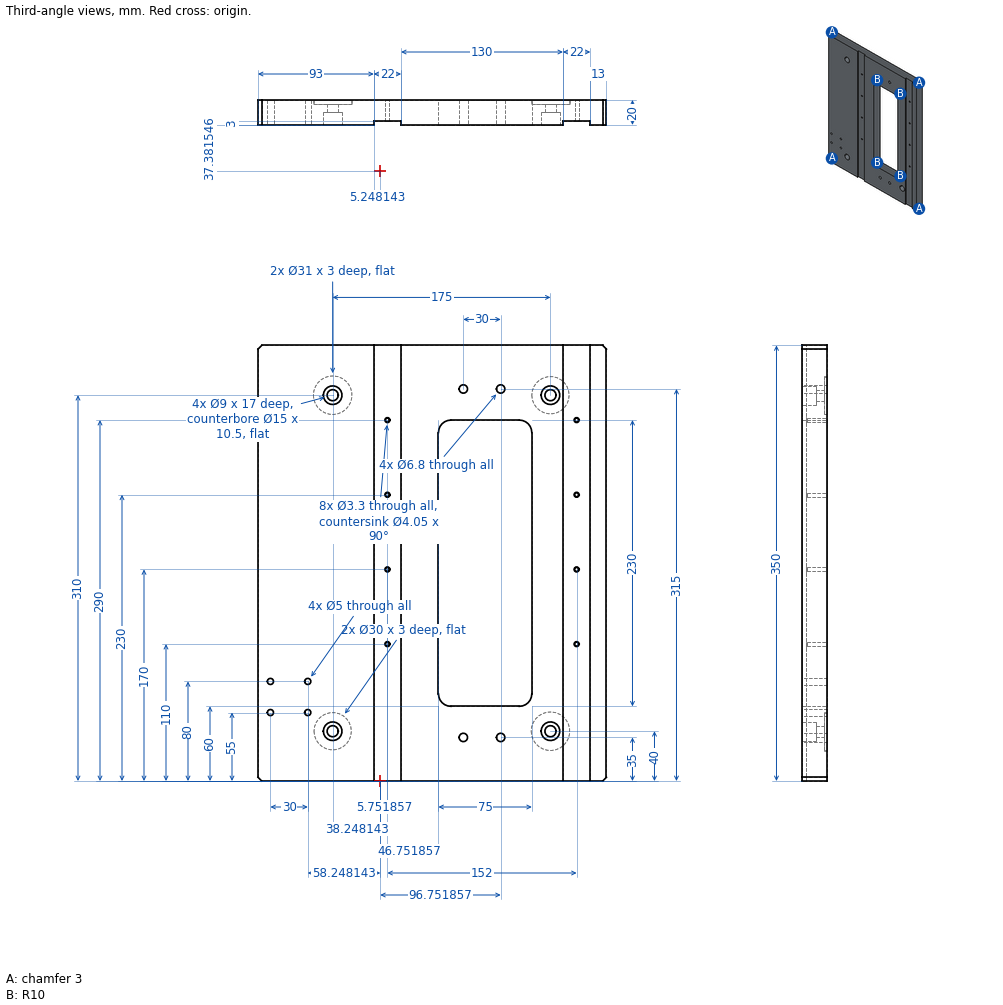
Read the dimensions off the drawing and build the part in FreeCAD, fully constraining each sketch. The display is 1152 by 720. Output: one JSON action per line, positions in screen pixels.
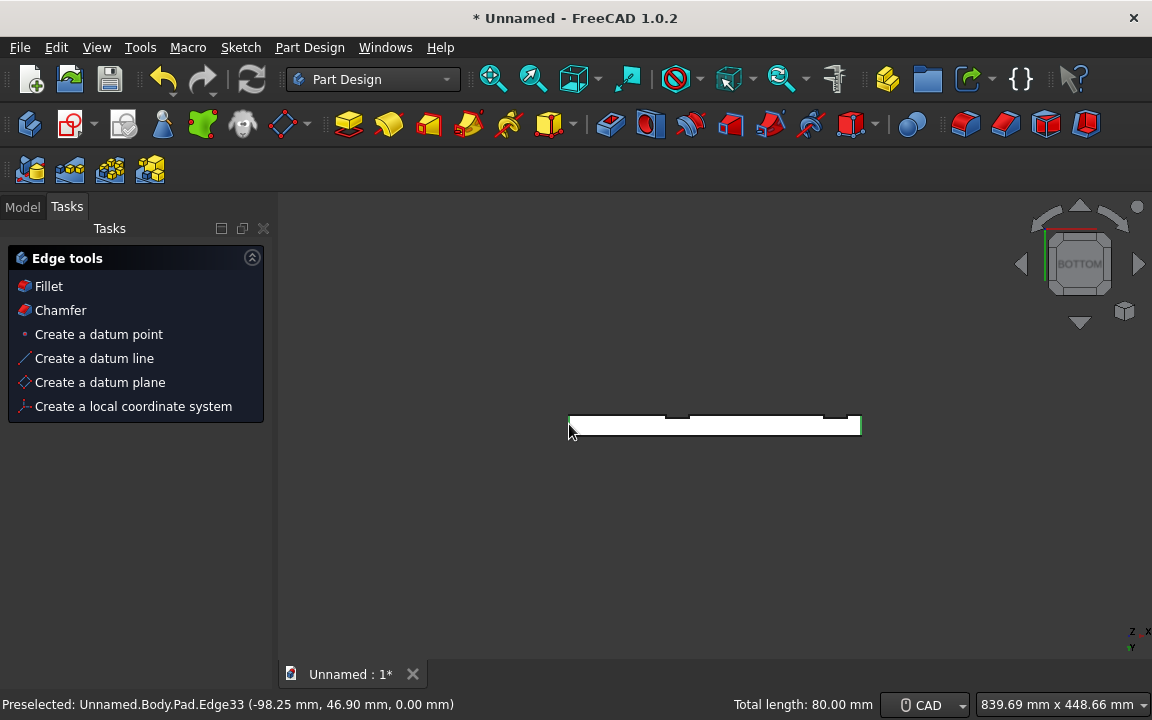
{"action": "left_click", "coordinate": [1006, 124]}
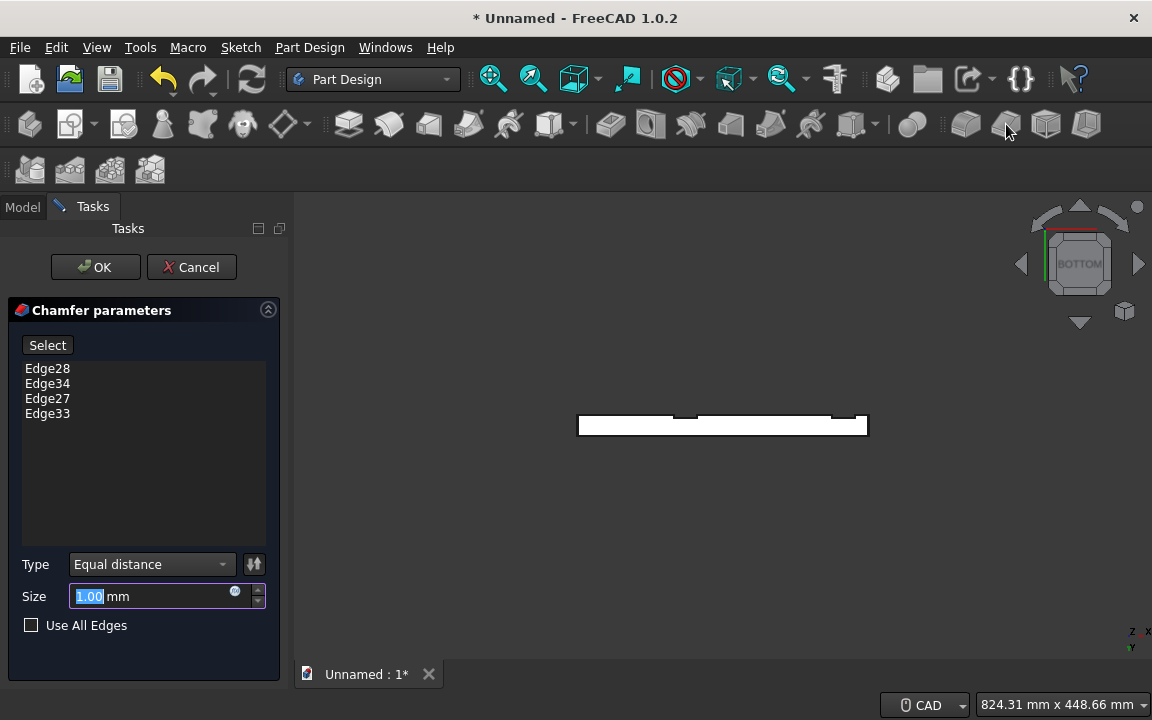
{"action": "type", "text": "3"}
{"action": "key", "text": "Tab"}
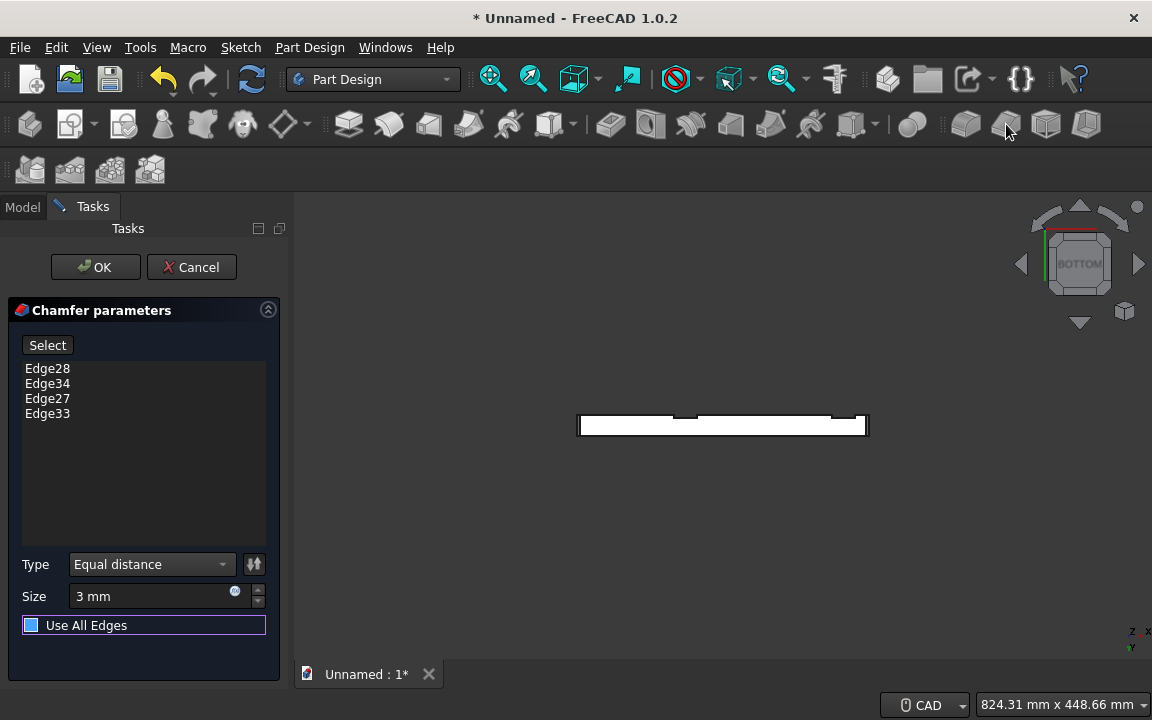
{"action": "left_click", "coordinate": [96, 267]}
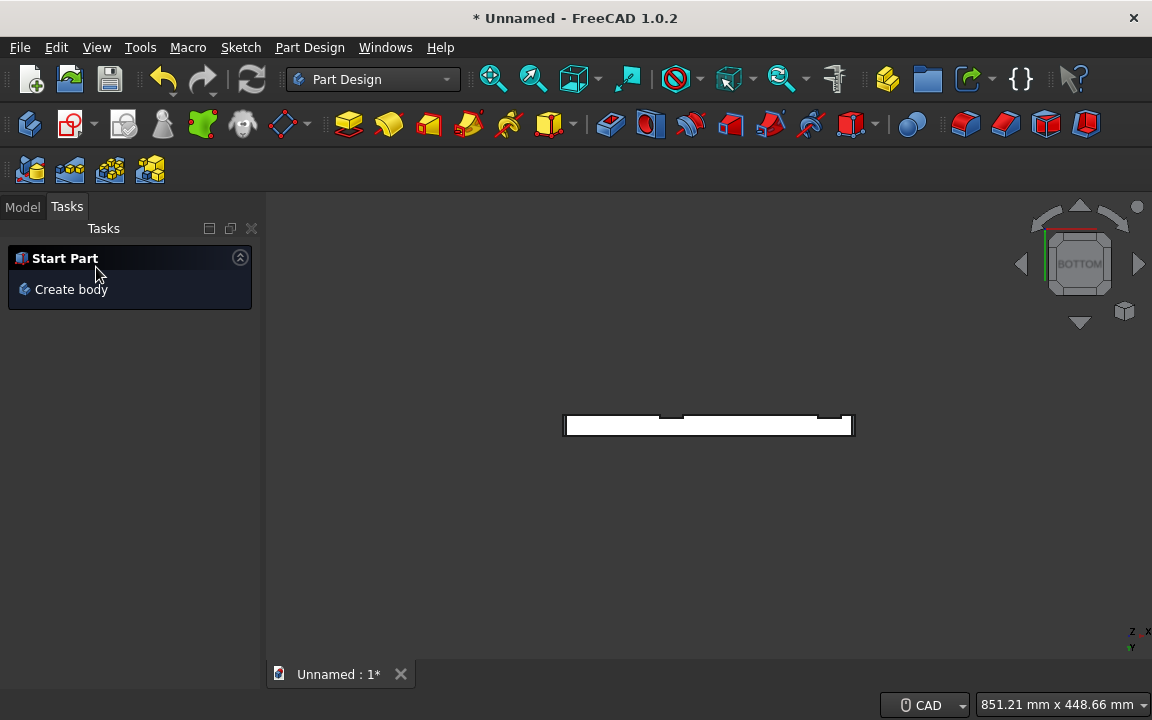
{"action": "left_click", "coordinate": [494, 80]}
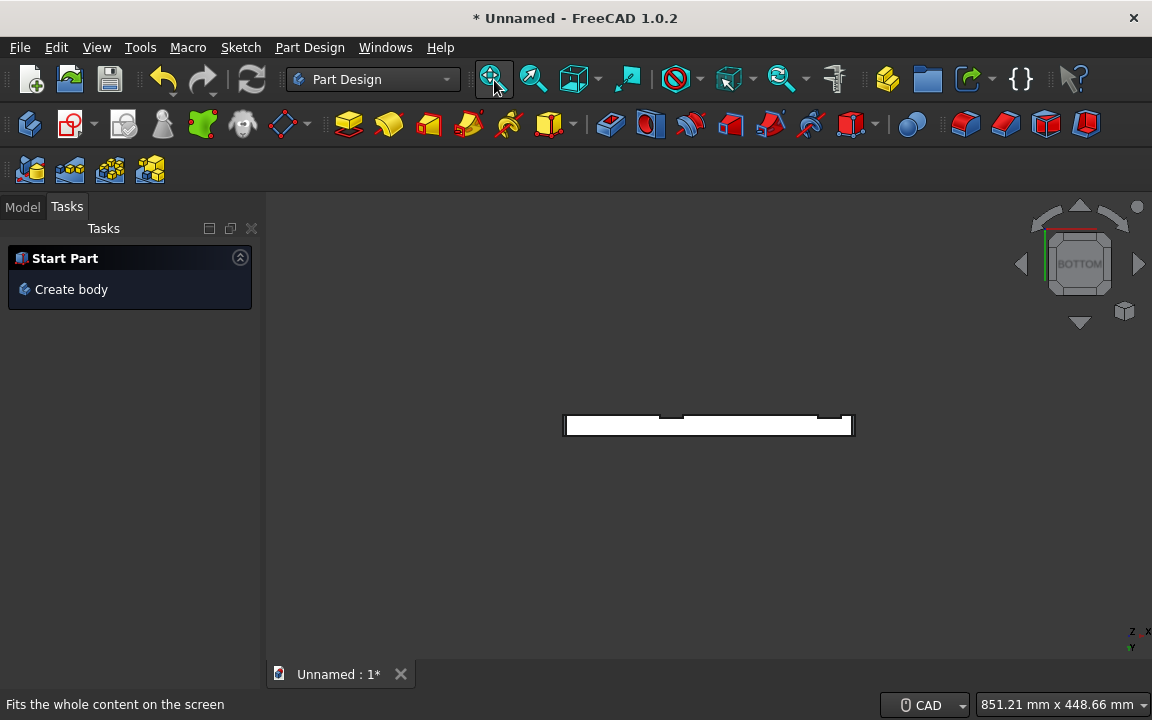
{"action": "key", "text": "0"}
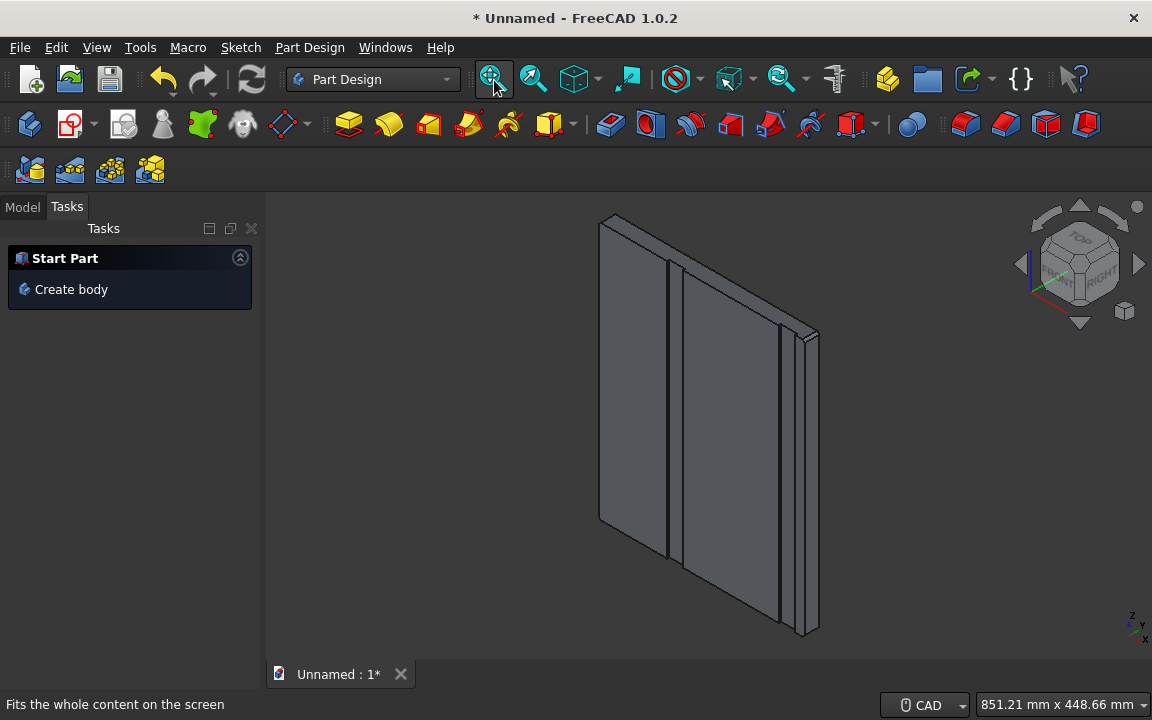
{"action": "left_click", "coordinate": [731, 361]}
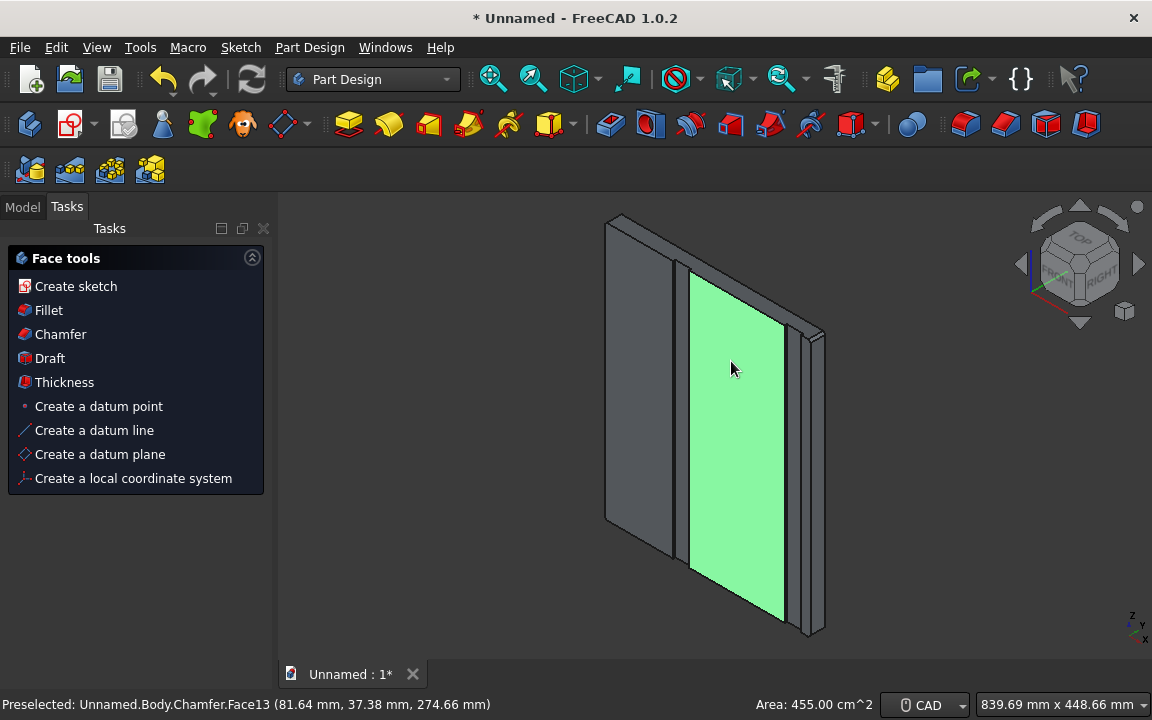
{"action": "left_click", "coordinate": [70, 124]}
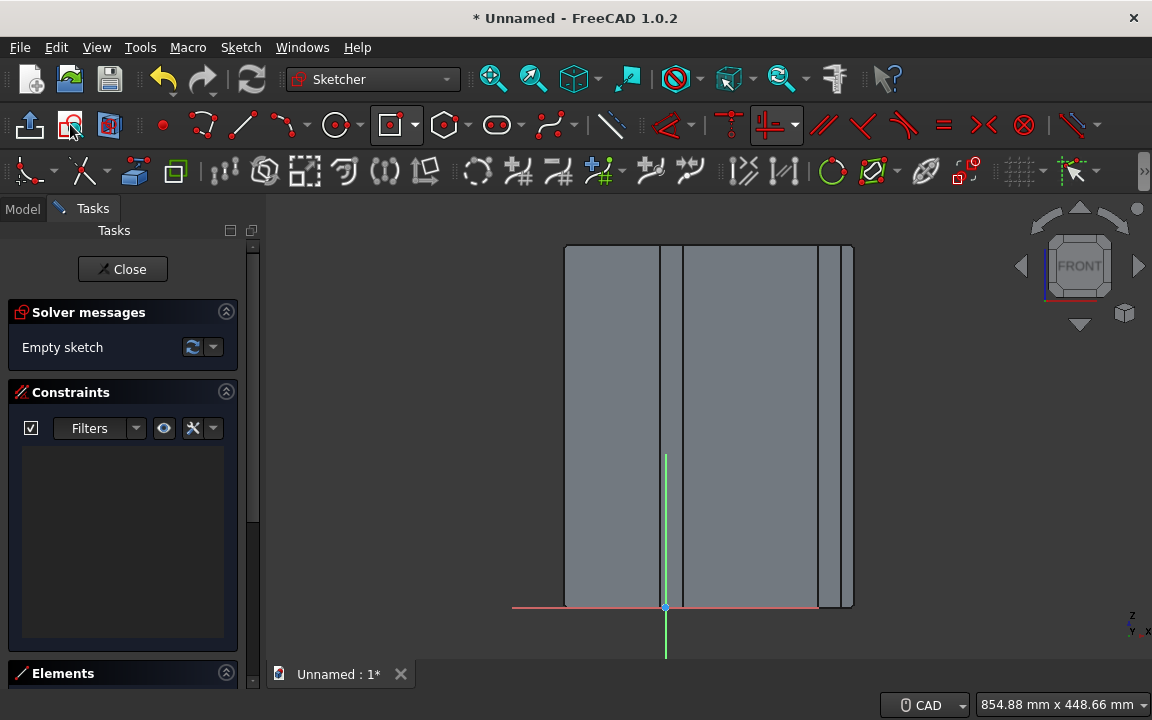
{"action": "scroll", "coordinate": [294, 286], "scroll_direction": "down", "scroll_amount": 1}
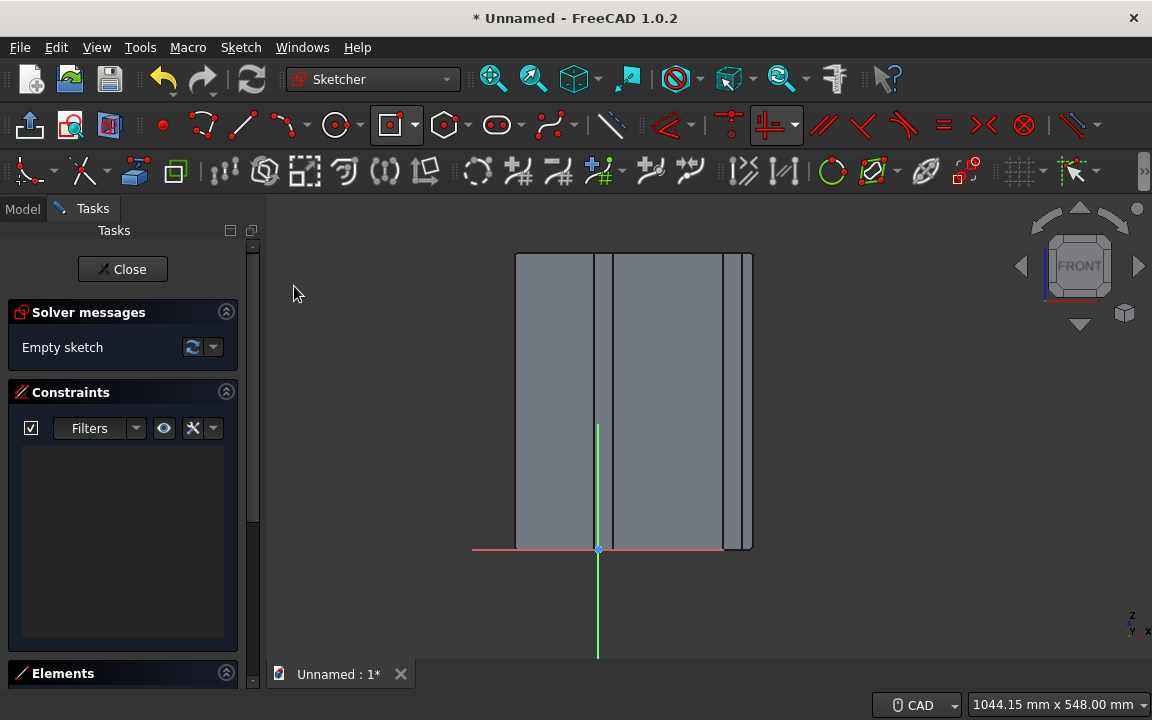
{"action": "left_click", "coordinate": [418, 126]}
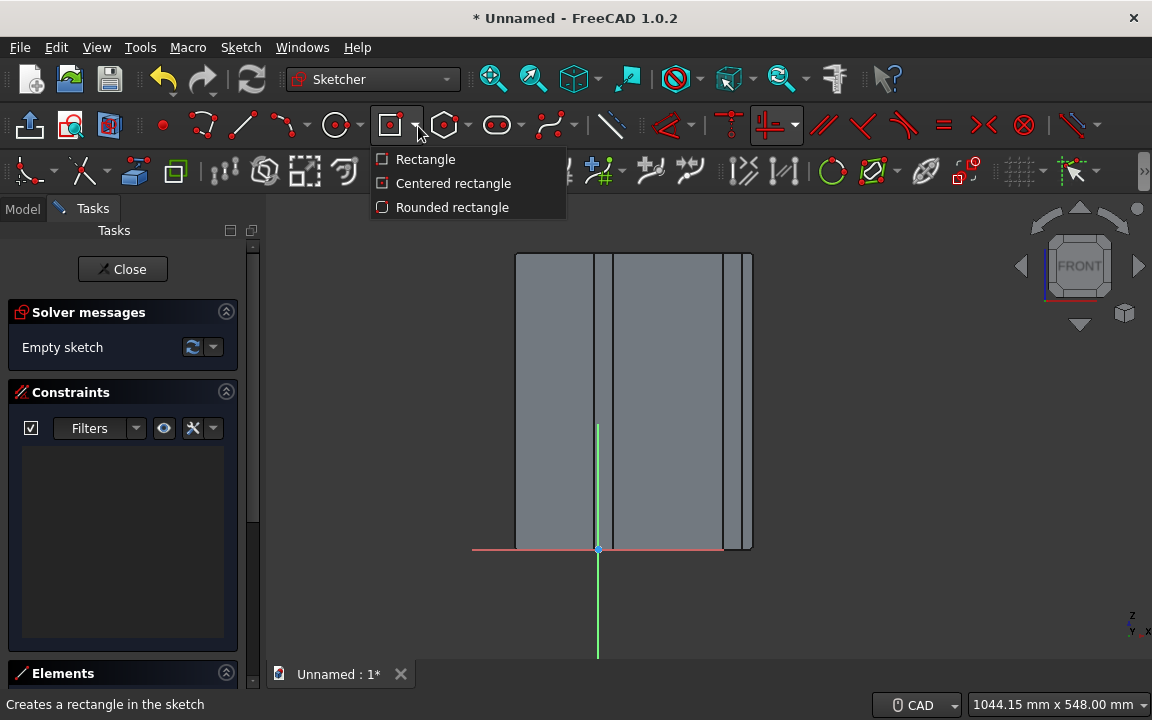
{"action": "left_click", "coordinate": [468, 159]}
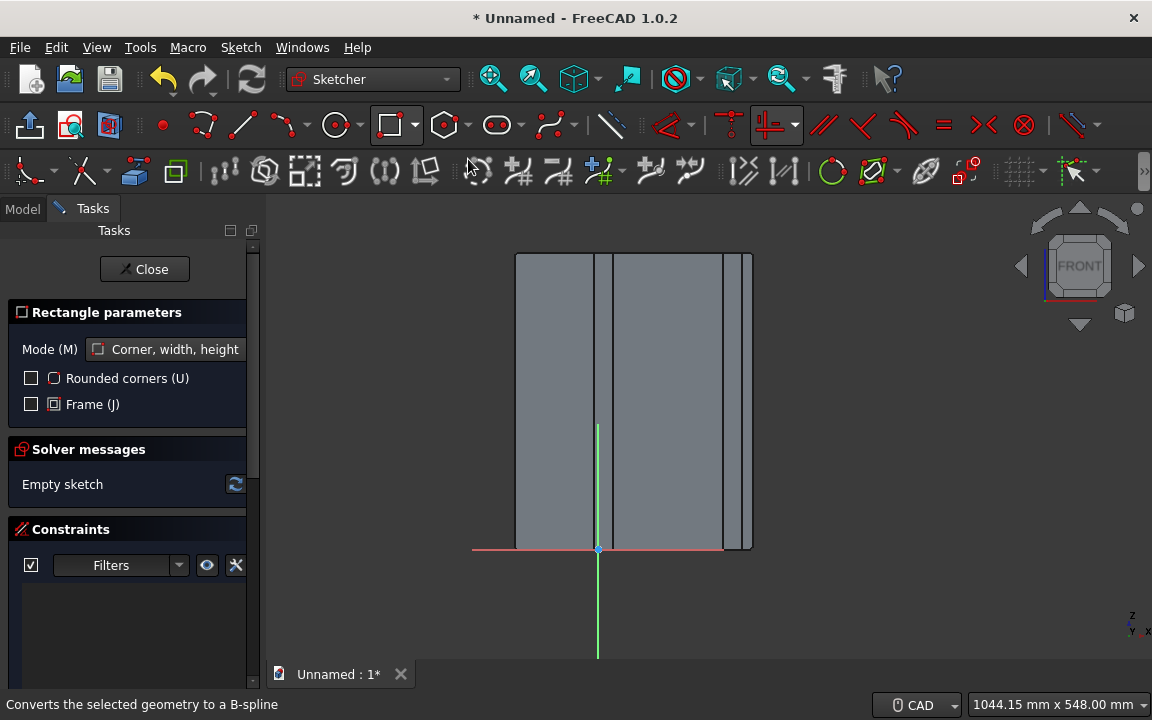
{"action": "left_click", "coordinate": [638, 303]}
{"action": "mouse_move", "coordinate": [702, 499]}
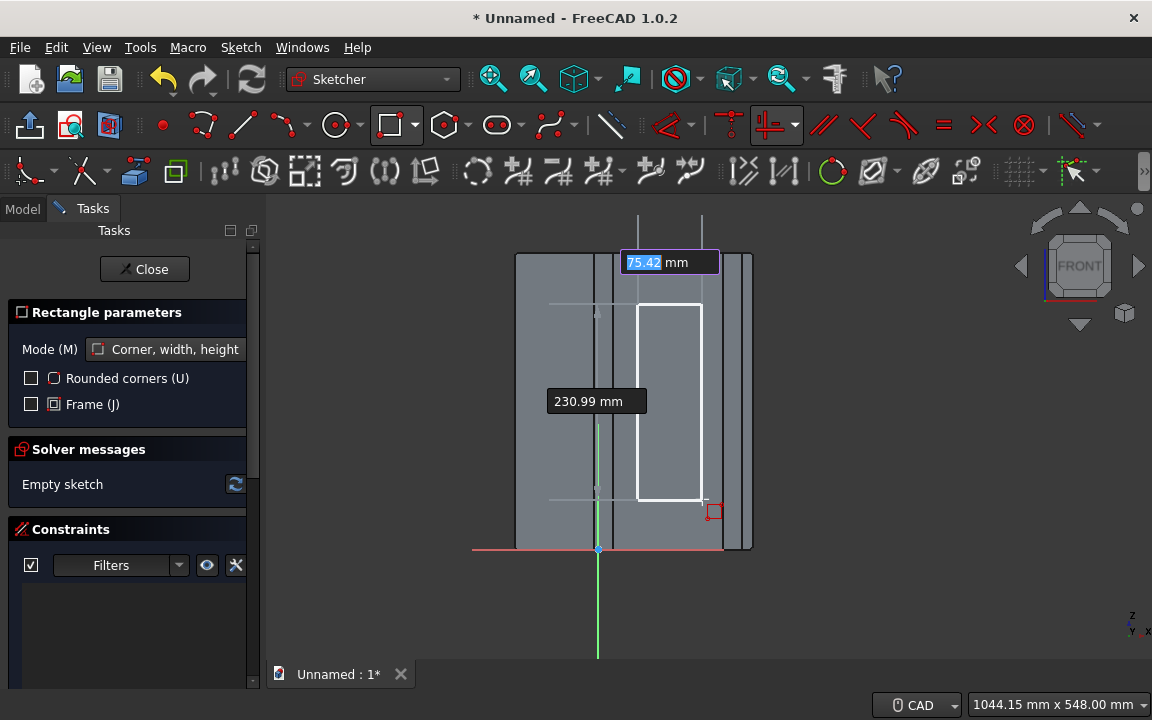
{"action": "type", "text": "75"}
{"action": "key", "text": "Tab"}
{"action": "type", "text": "230"}
{"action": "key", "text": "Return"}
{"action": "key", "text": "Escape"}